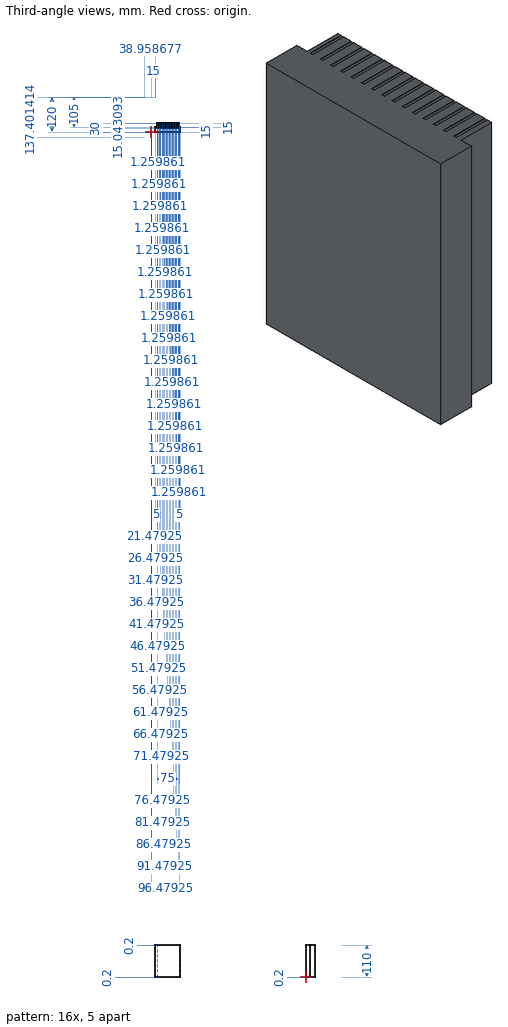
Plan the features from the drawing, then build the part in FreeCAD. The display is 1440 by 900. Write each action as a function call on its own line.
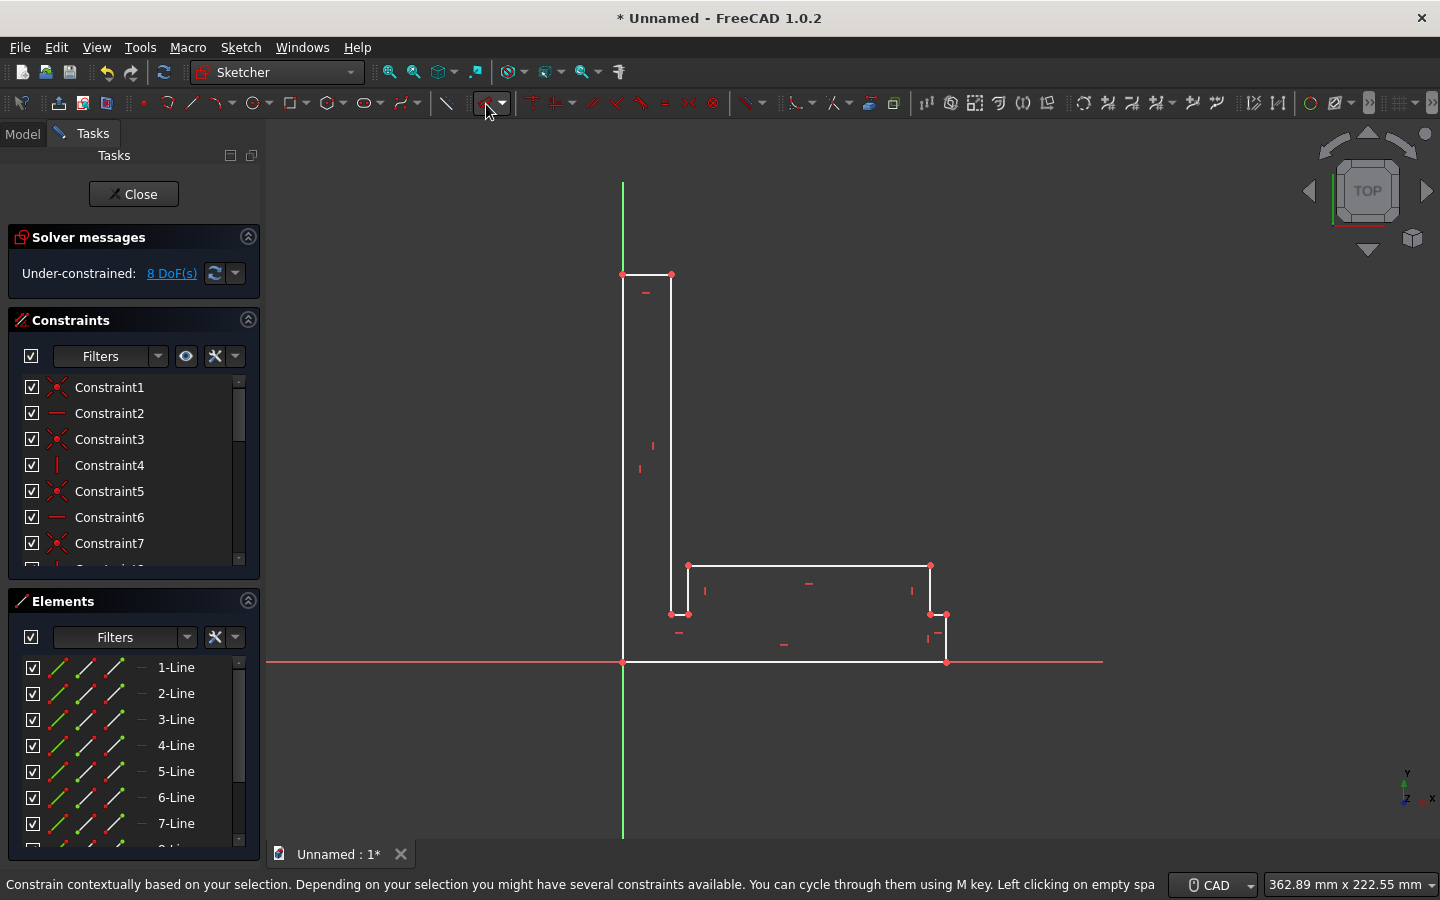
scroll(938, 615, up, 5)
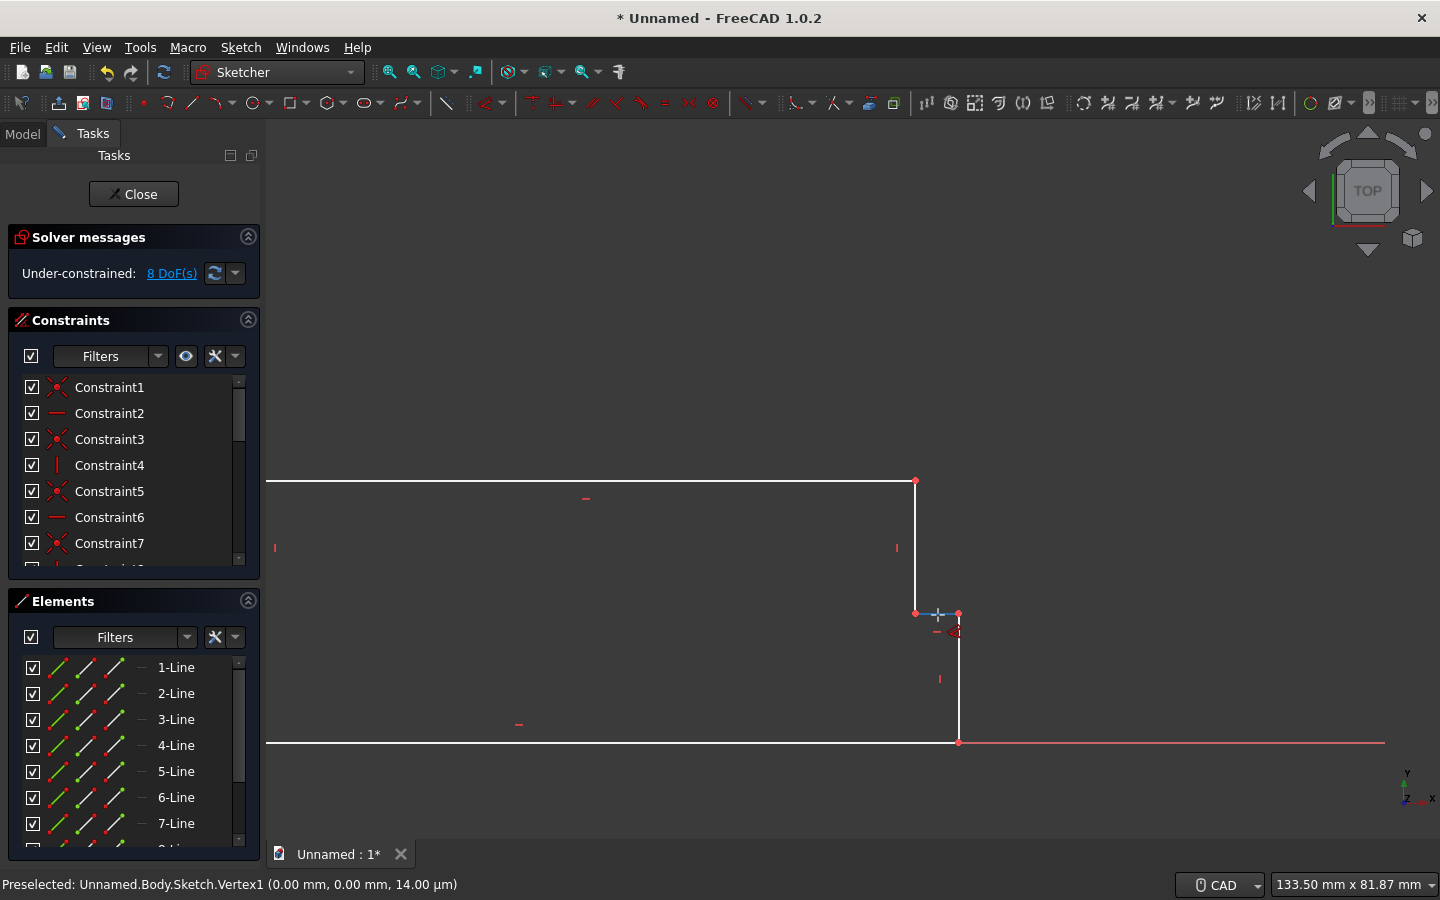
click(937, 614)
click(937, 648)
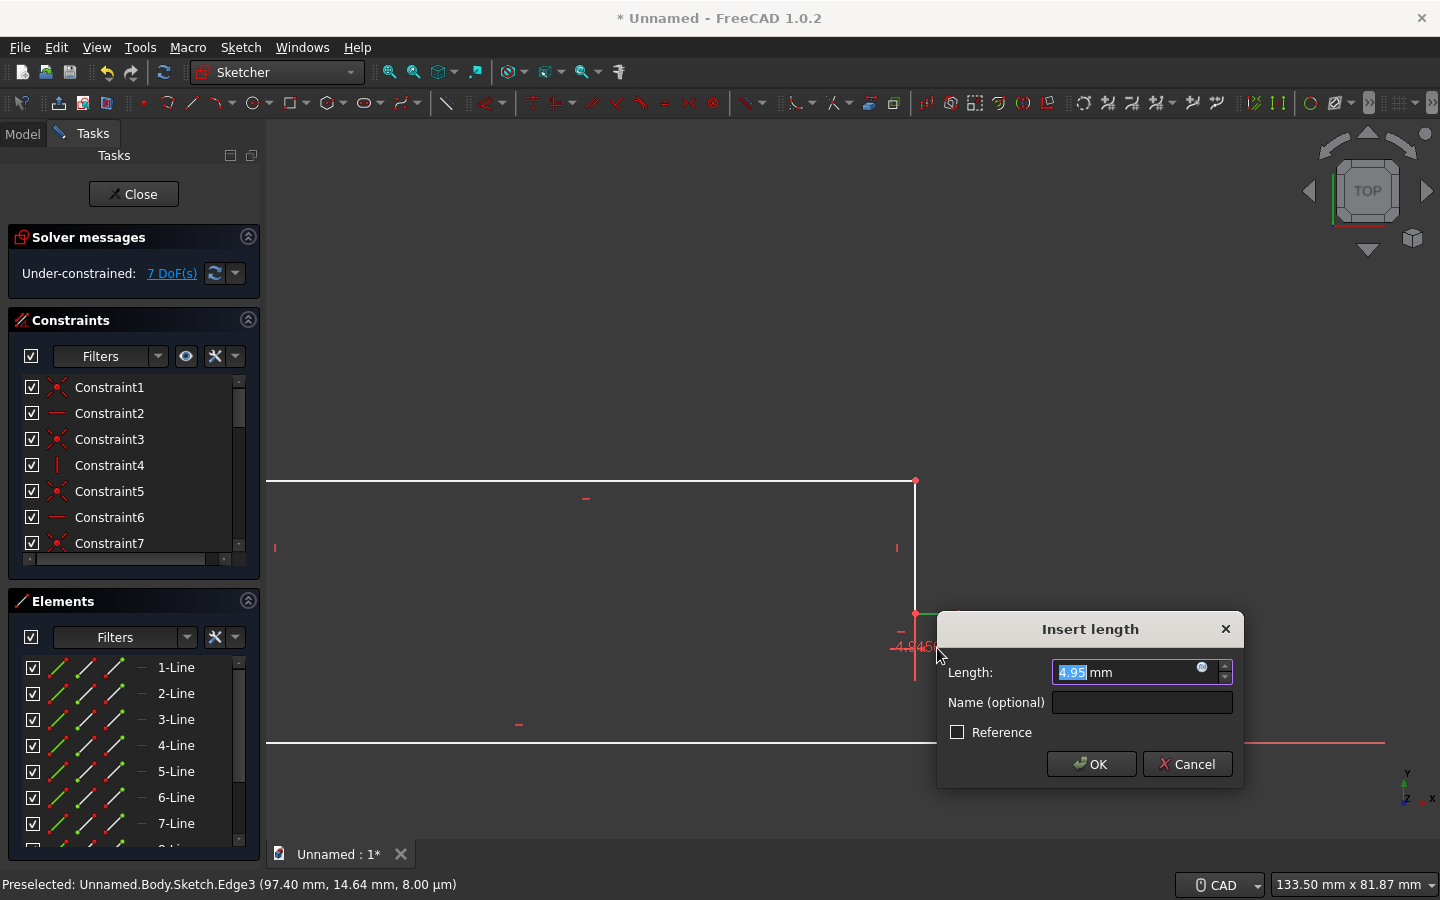
text(5)
key(Return)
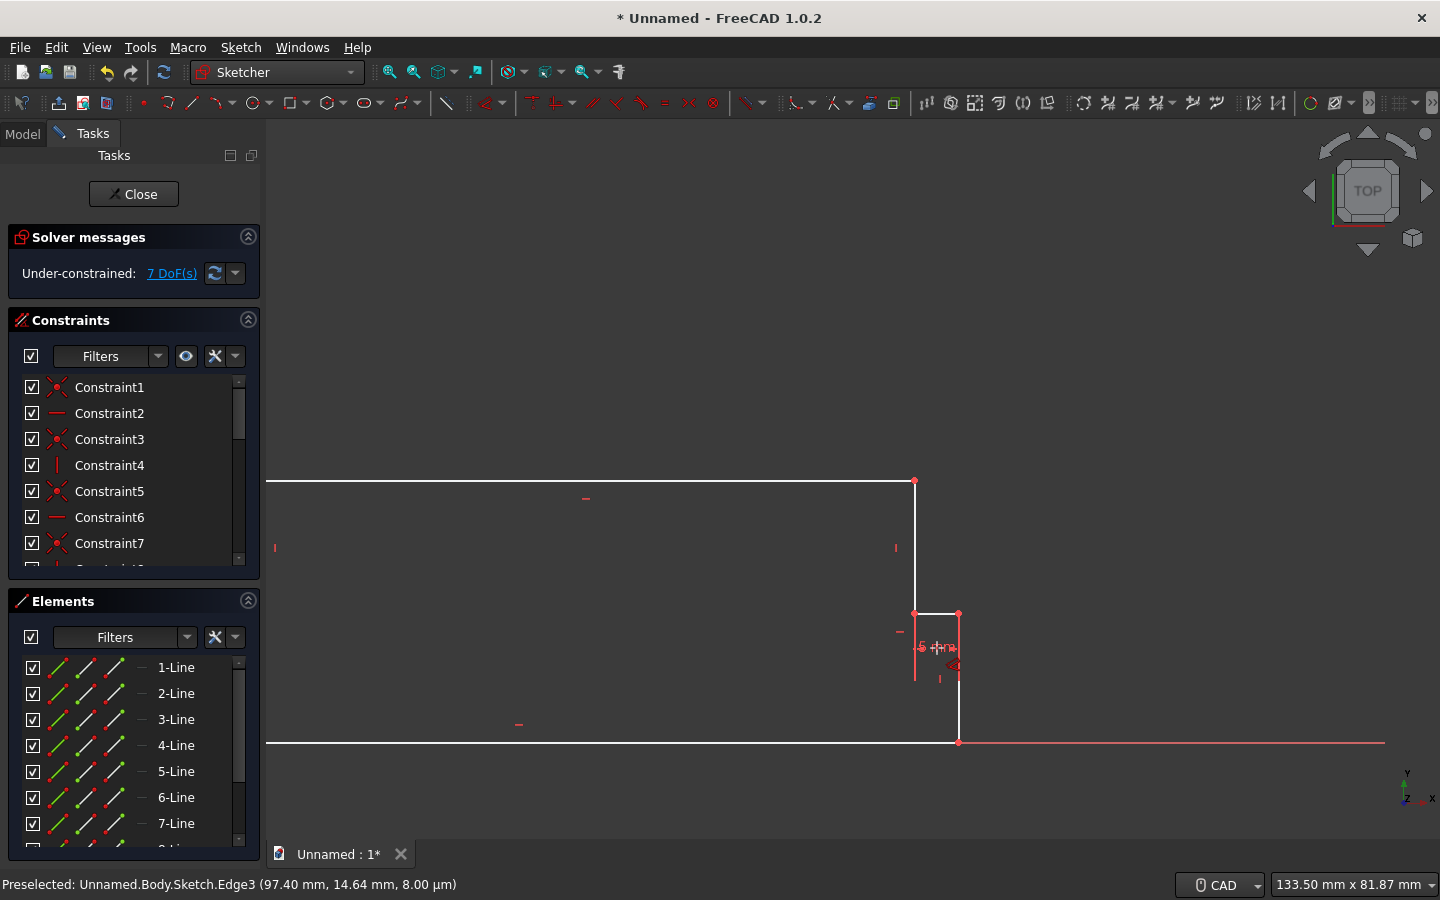
scroll(1000, 695, down, 4)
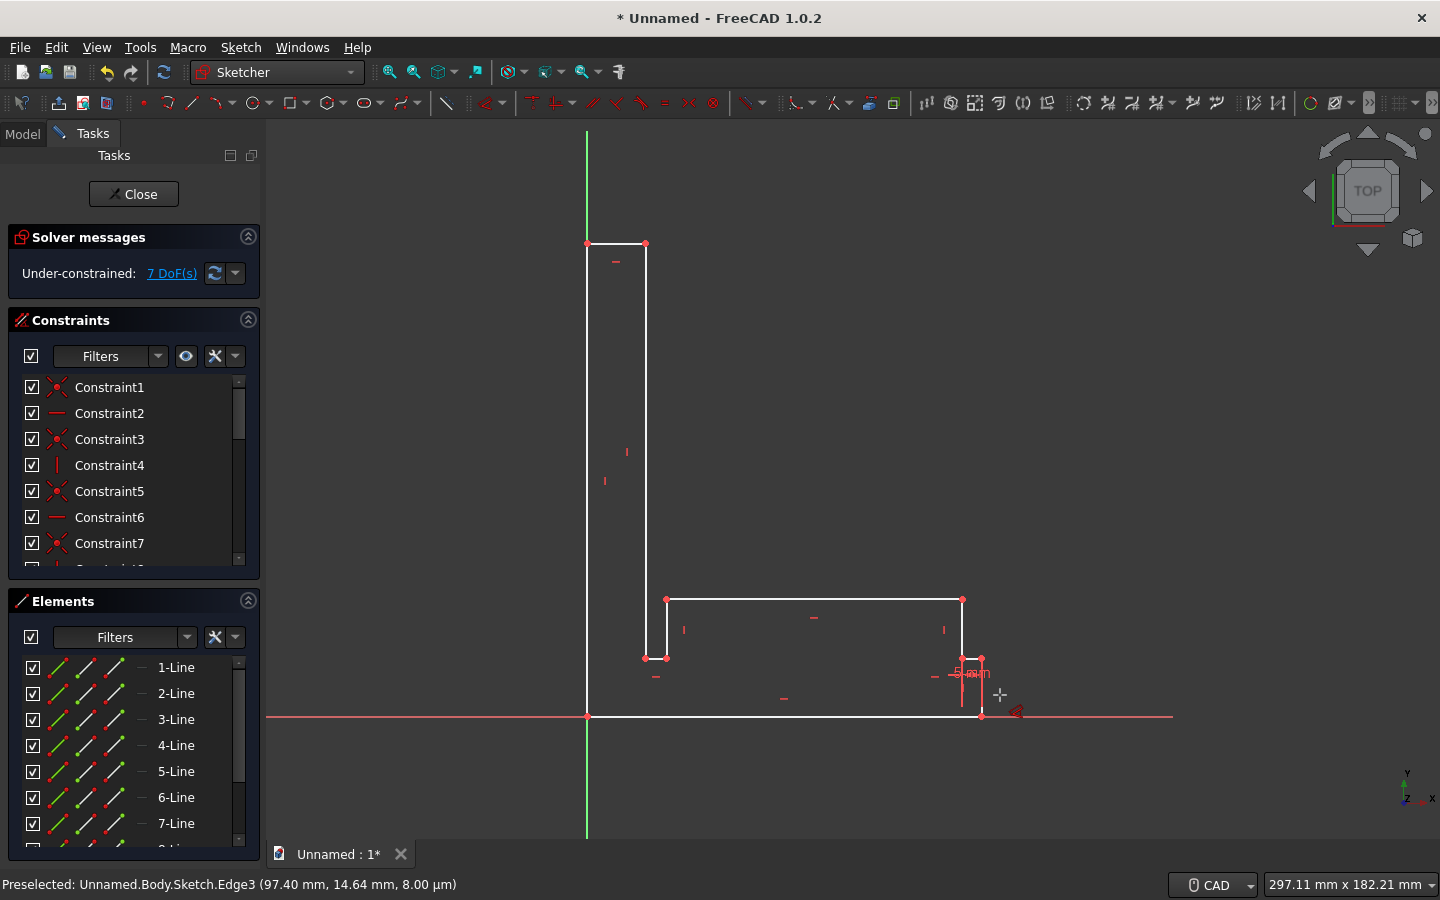
scroll(660, 659, up, 4)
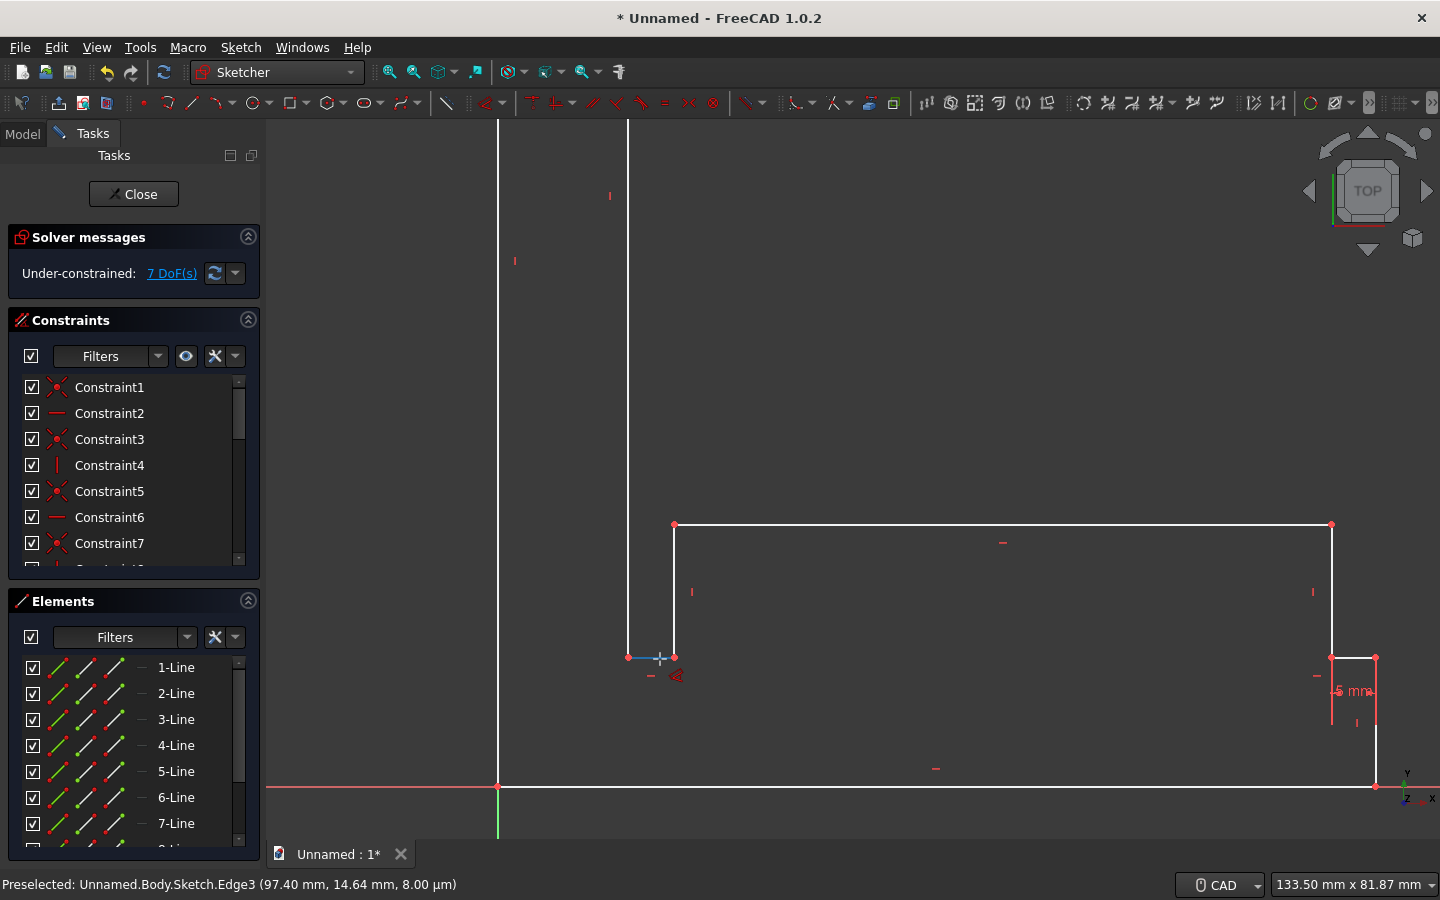
click(661, 658)
click(651, 692)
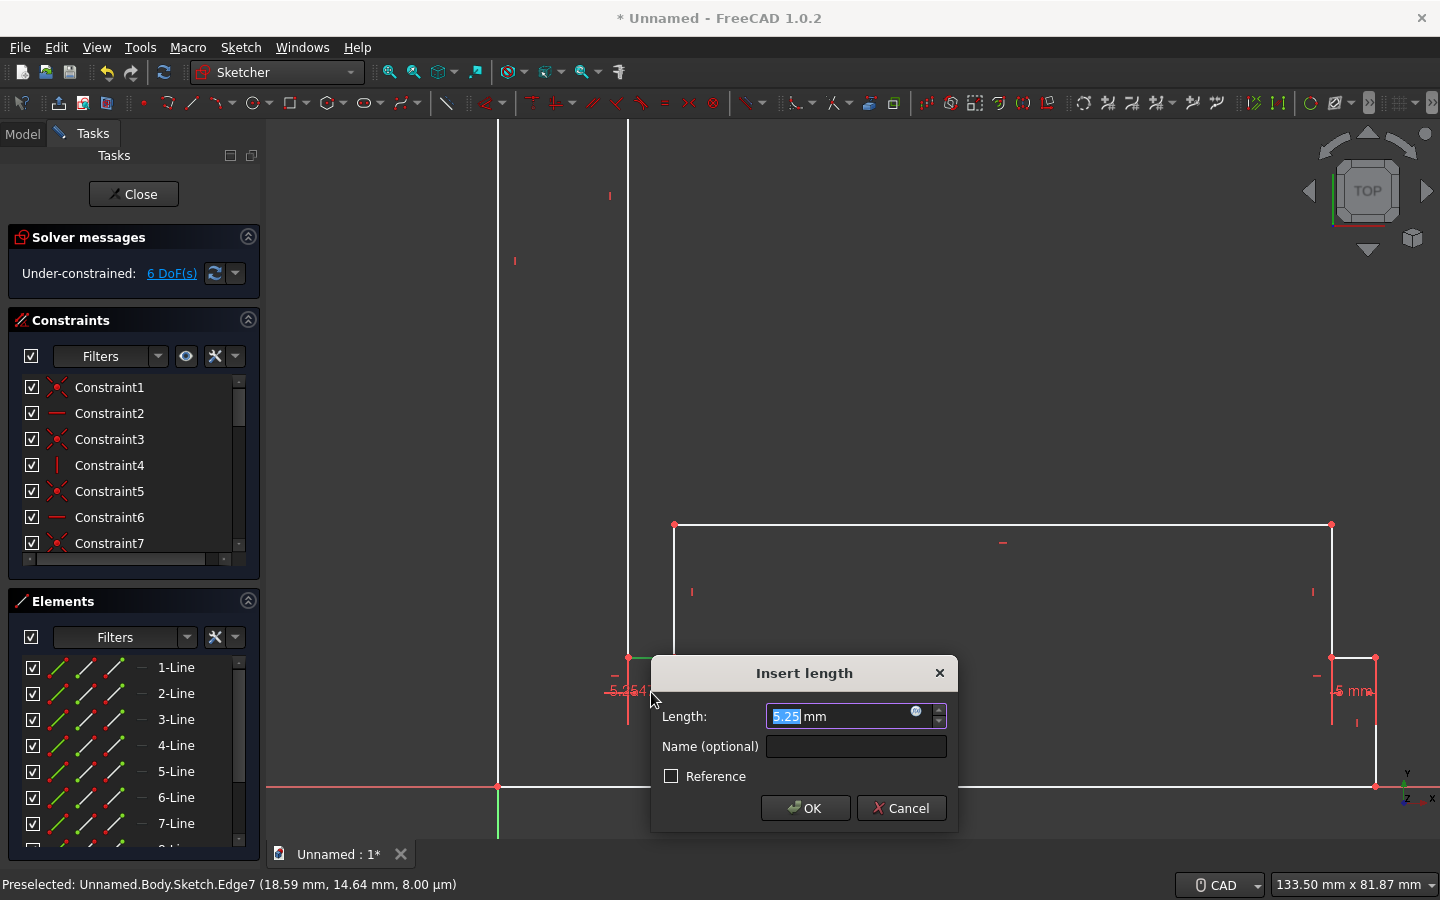
text(5)
key(Return)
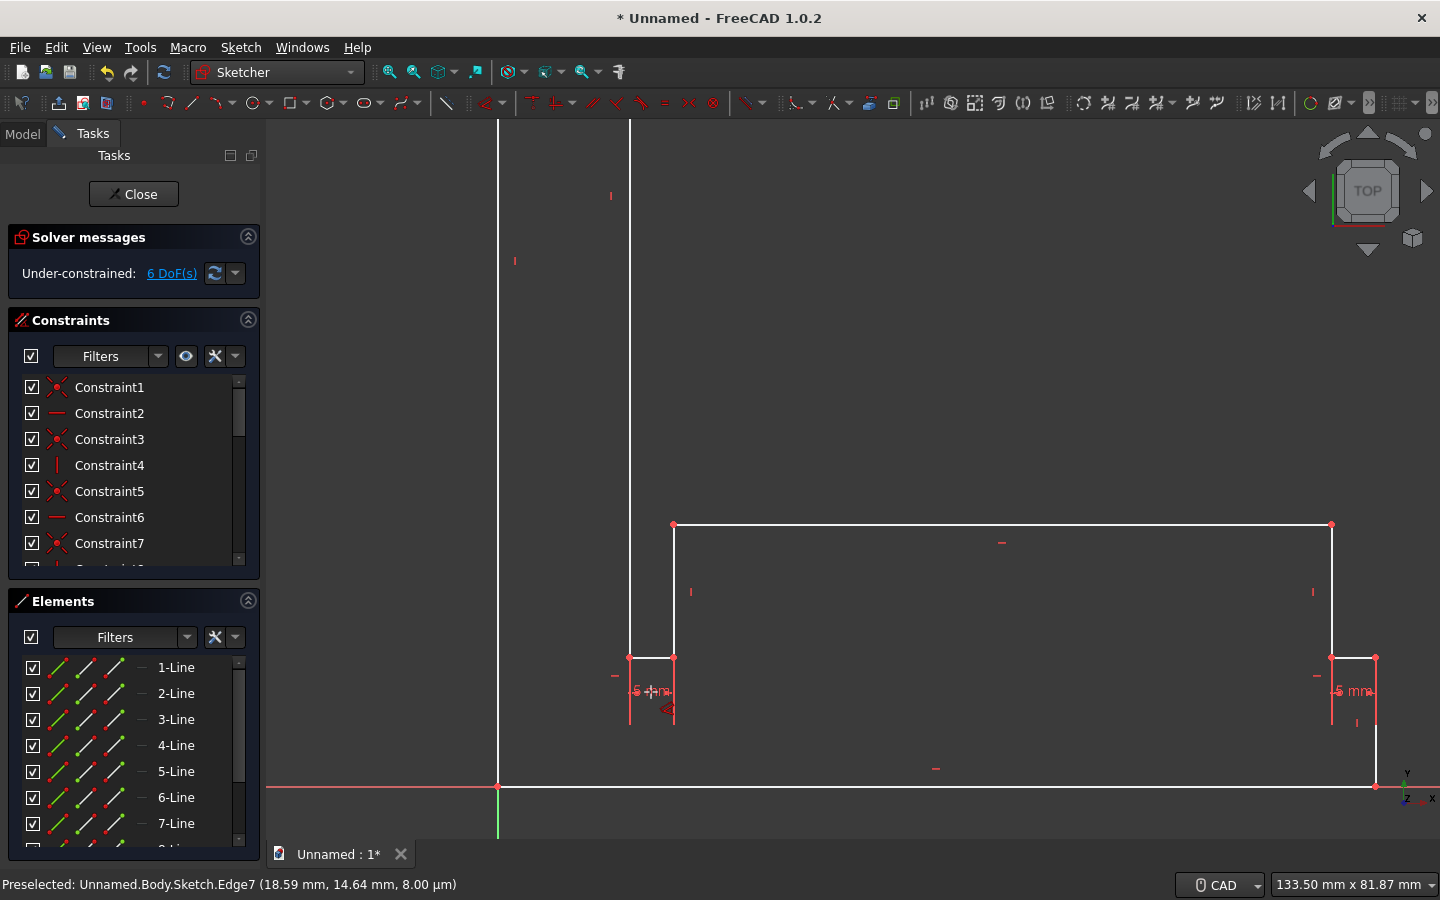
scroll(660, 658, down, 4)